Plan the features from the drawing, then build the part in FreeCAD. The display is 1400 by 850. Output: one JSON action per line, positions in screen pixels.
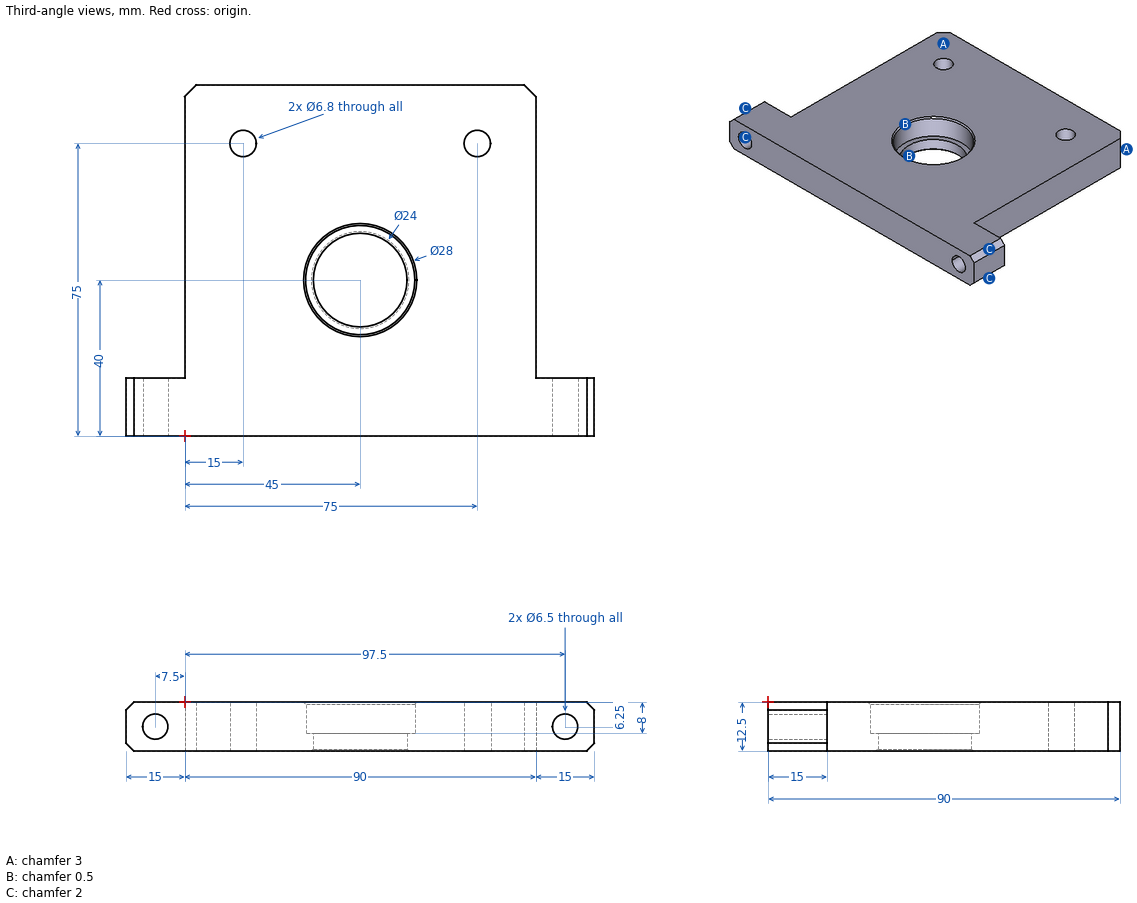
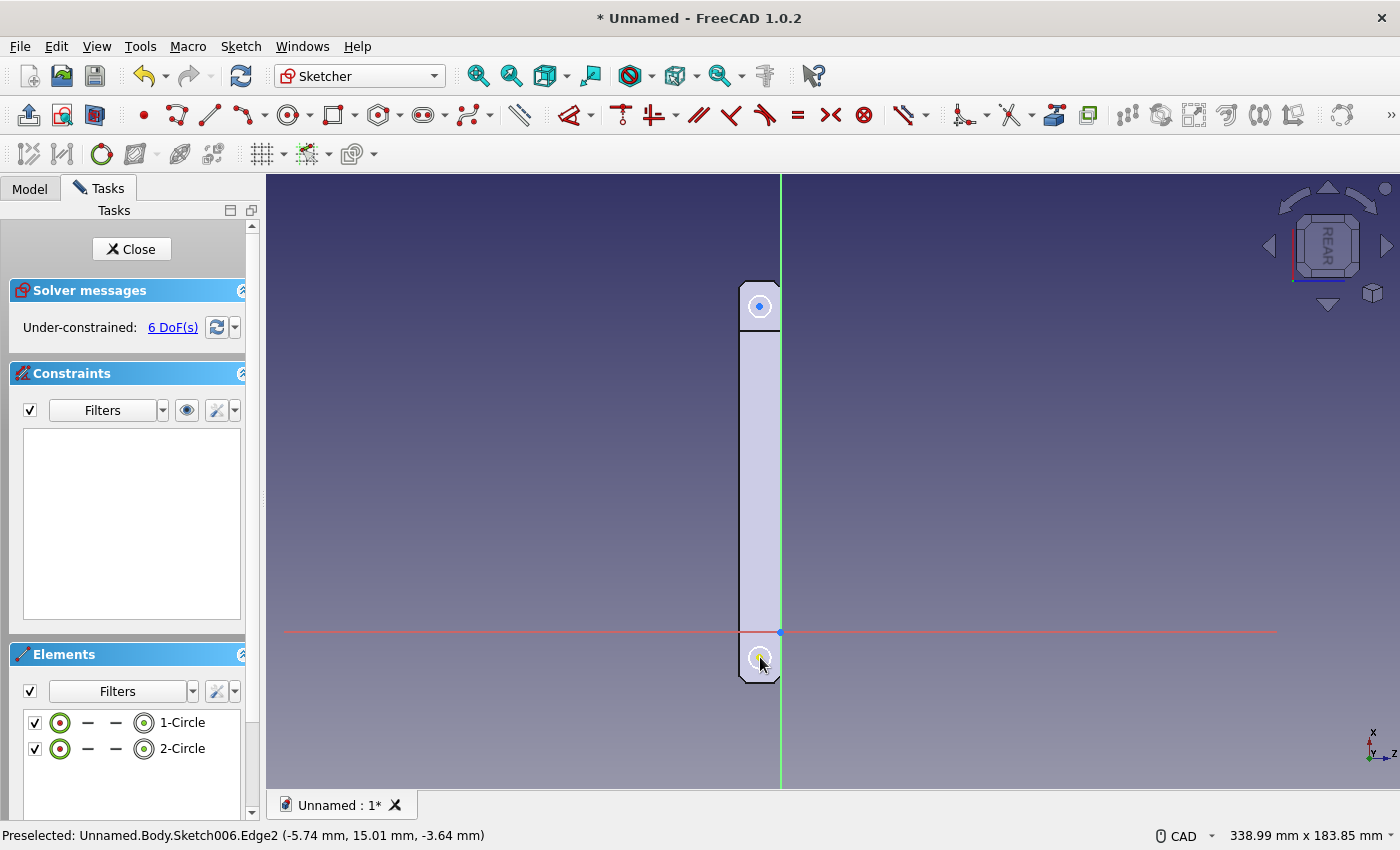
{"action": "scroll", "coordinate": [768, 299], "scroll_direction": "up", "scroll_amount": 2}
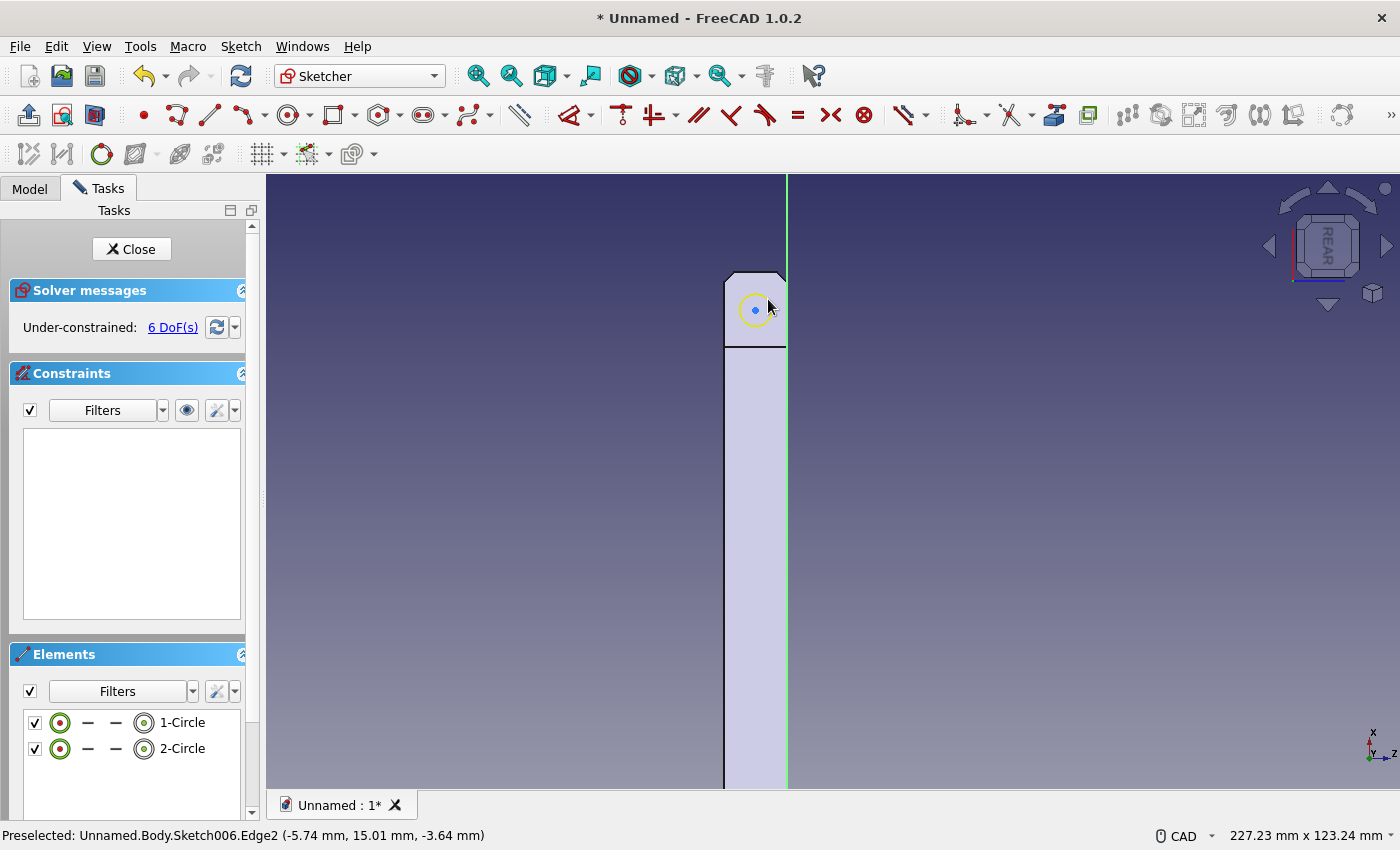
{"action": "left_click", "coordinate": [767, 299]}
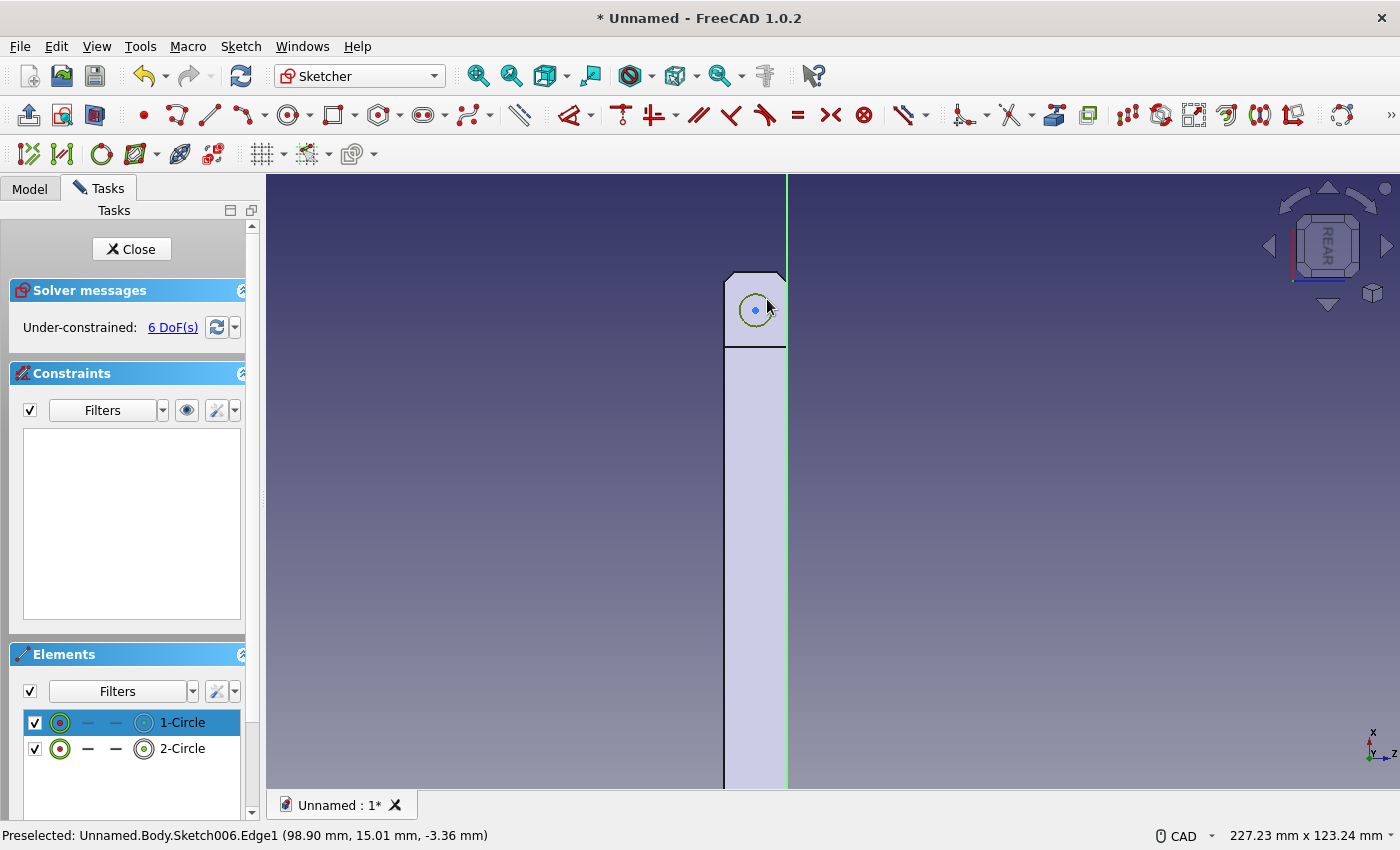
{"action": "scroll", "coordinate": [768, 298], "scroll_direction": "down", "scroll_amount": 2}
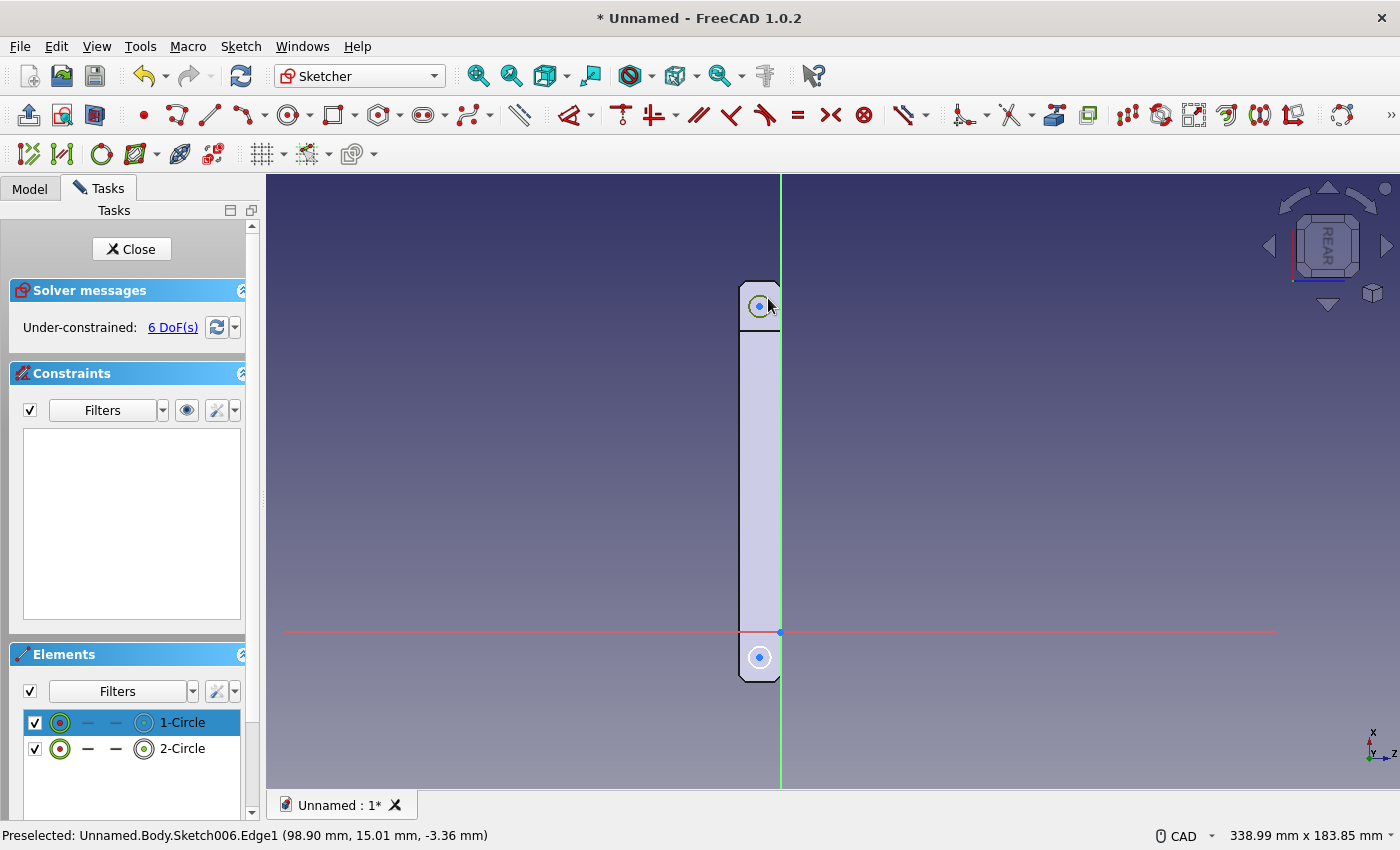
{"action": "scroll", "coordinate": [767, 650], "scroll_direction": "up", "scroll_amount": 2}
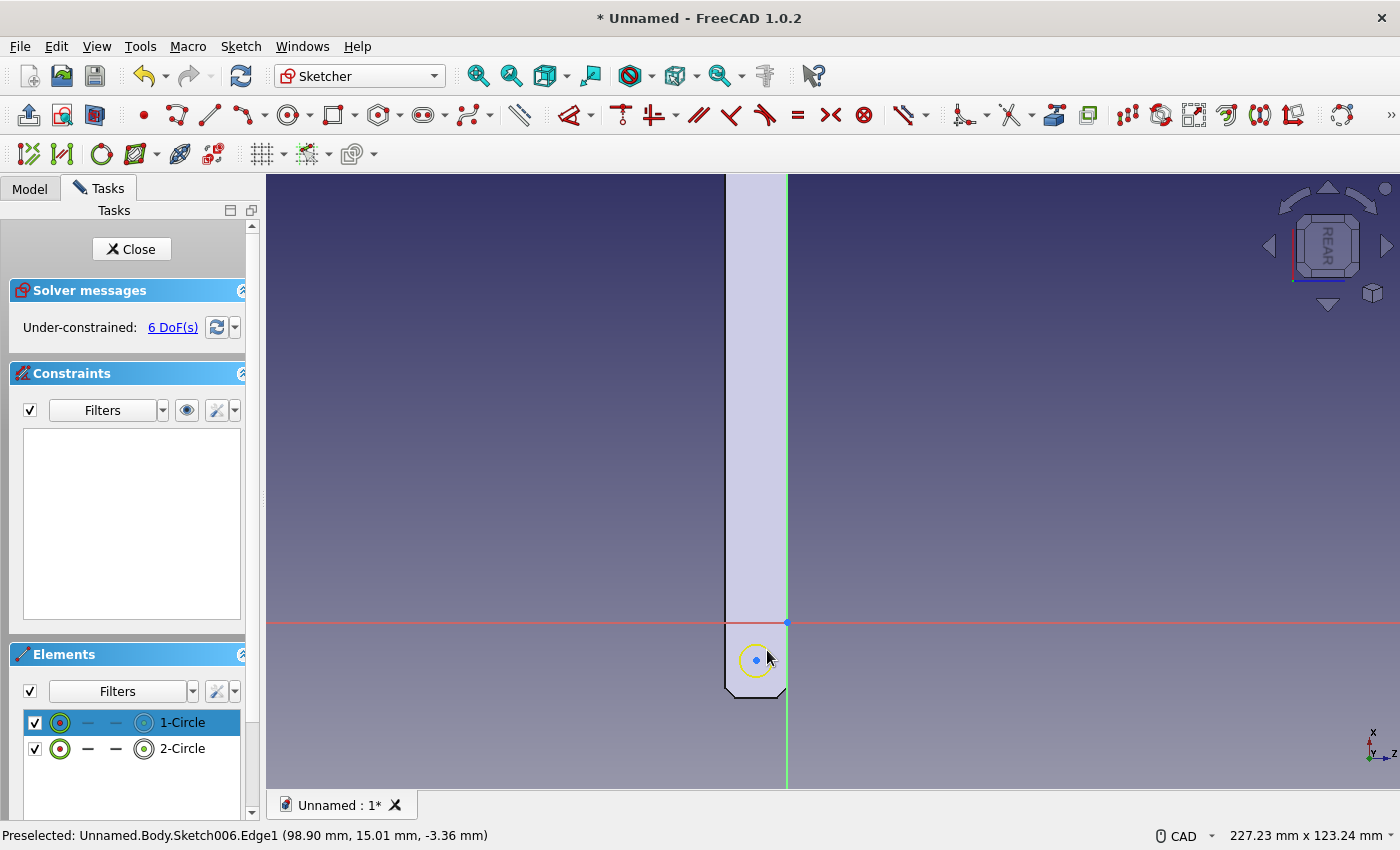
{"action": "left_click", "coordinate": [767, 649]}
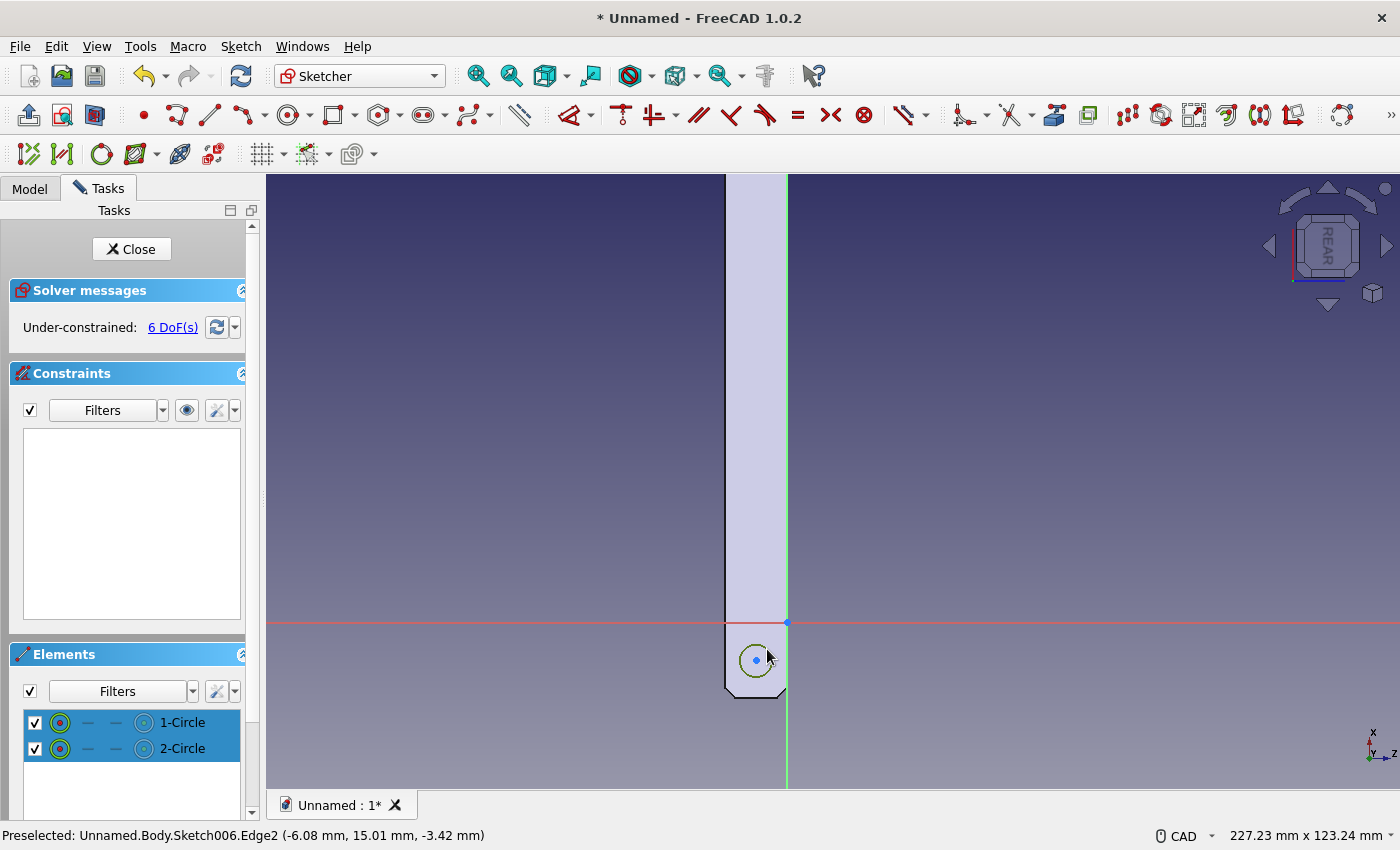
{"action": "left_click", "coordinate": [798, 116]}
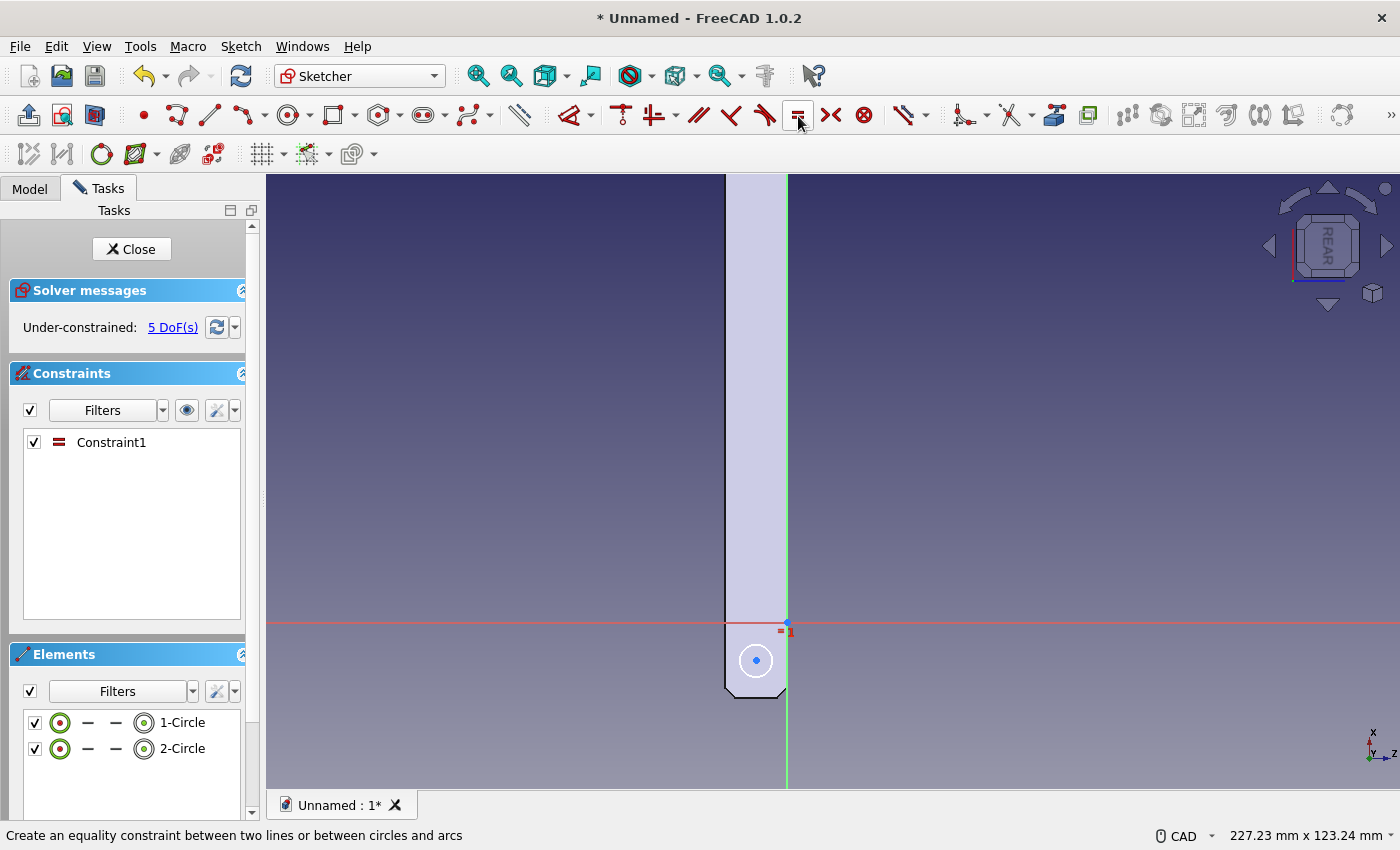
{"action": "left_click", "coordinate": [568, 116]}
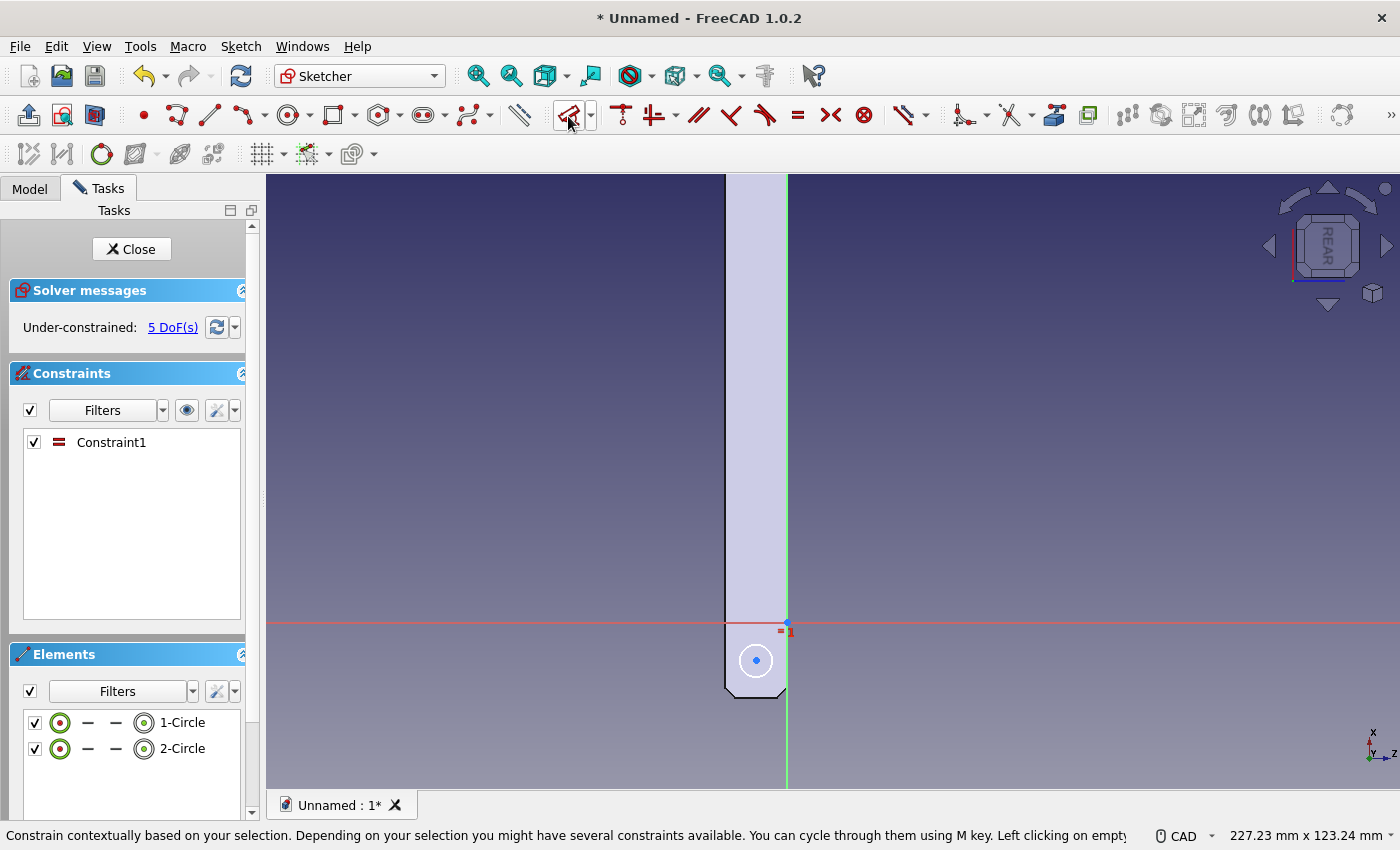
{"action": "scroll", "coordinate": [767, 651], "scroll_direction": "down", "scroll_amount": 2}